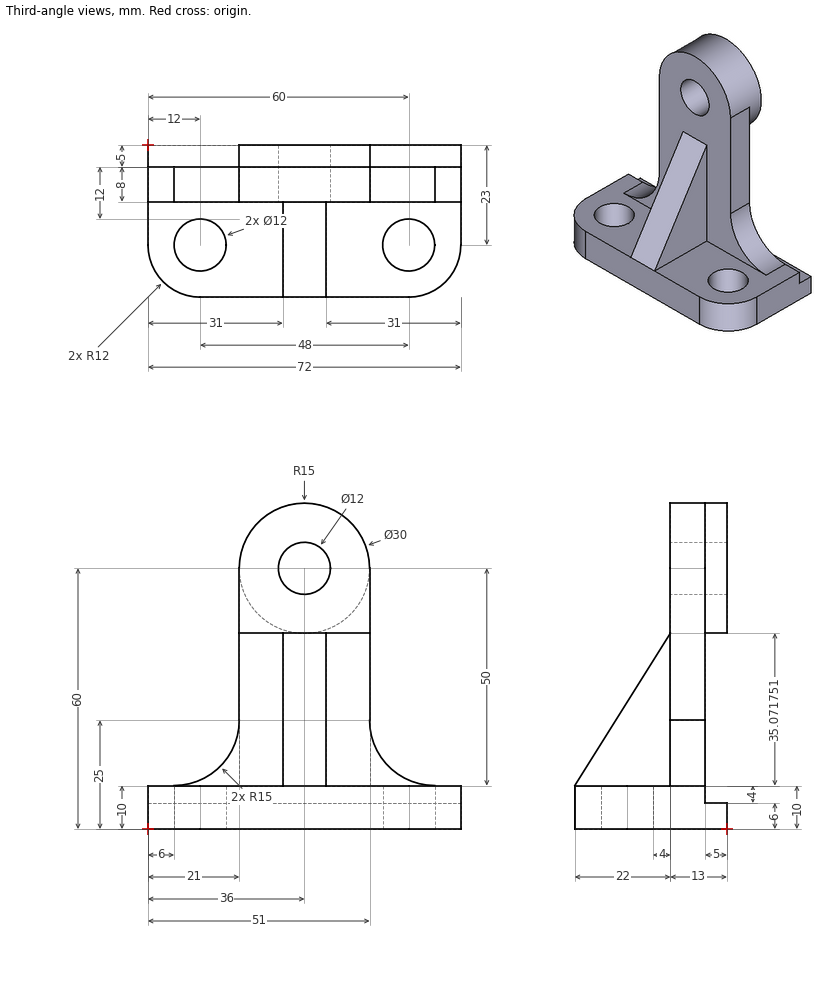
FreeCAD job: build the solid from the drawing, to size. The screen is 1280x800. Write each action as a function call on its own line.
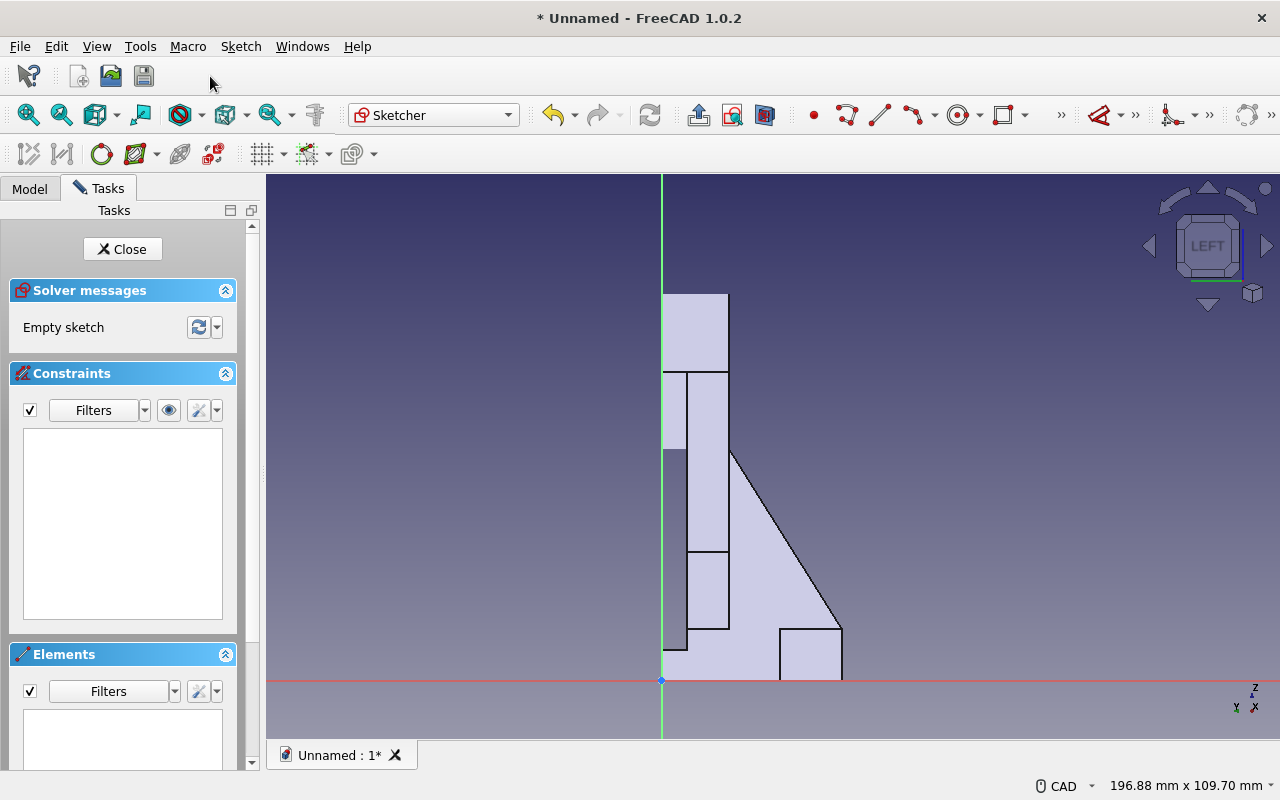
scroll(848, 711, up, 2)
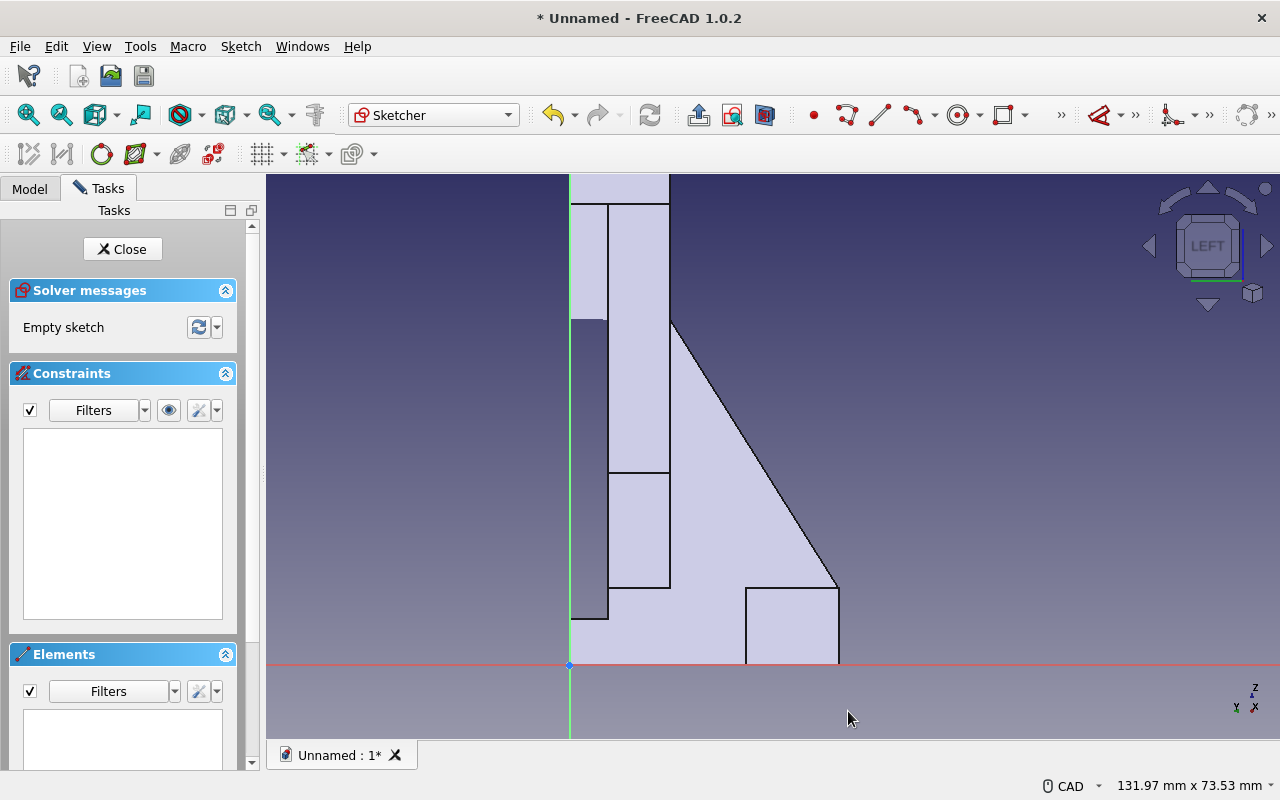
click(847, 116)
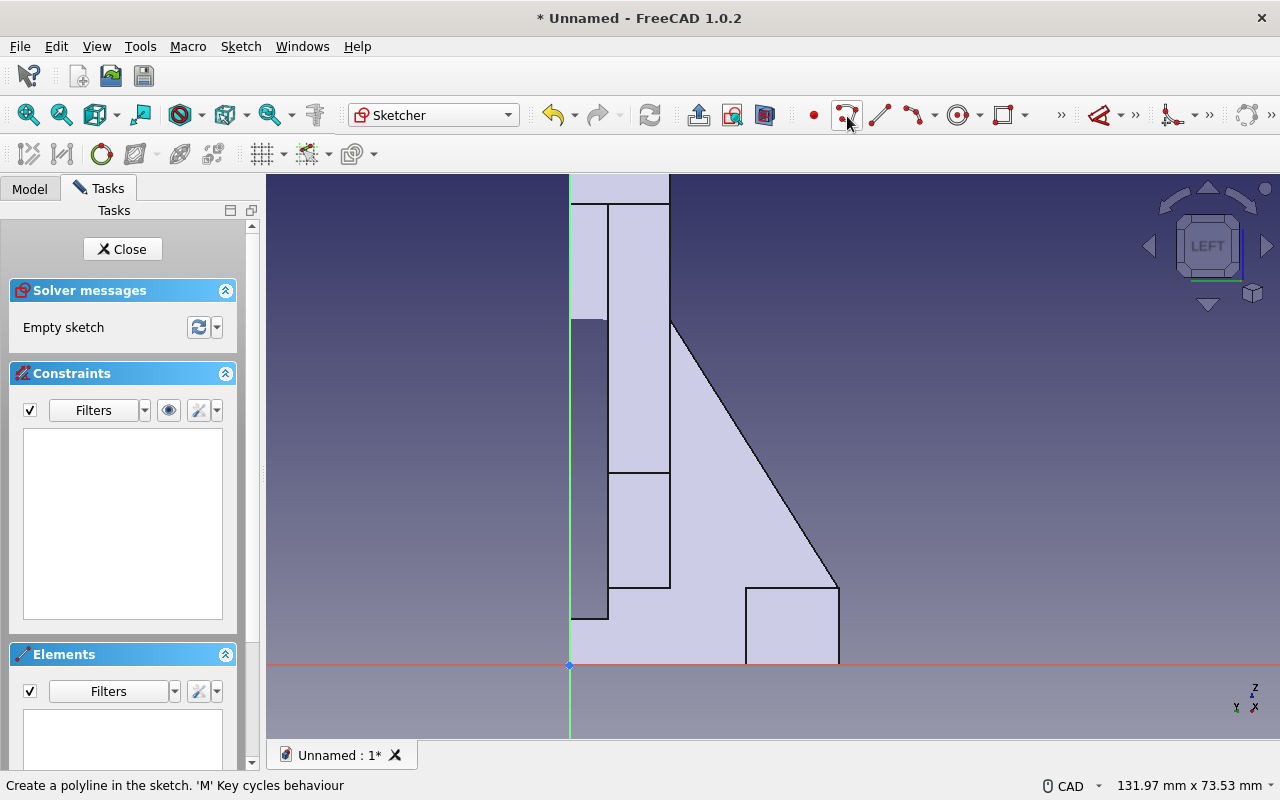
click(670, 588)
click(839, 588)
click(670, 319)
click(670, 589)
key(Escape)
key(Escape)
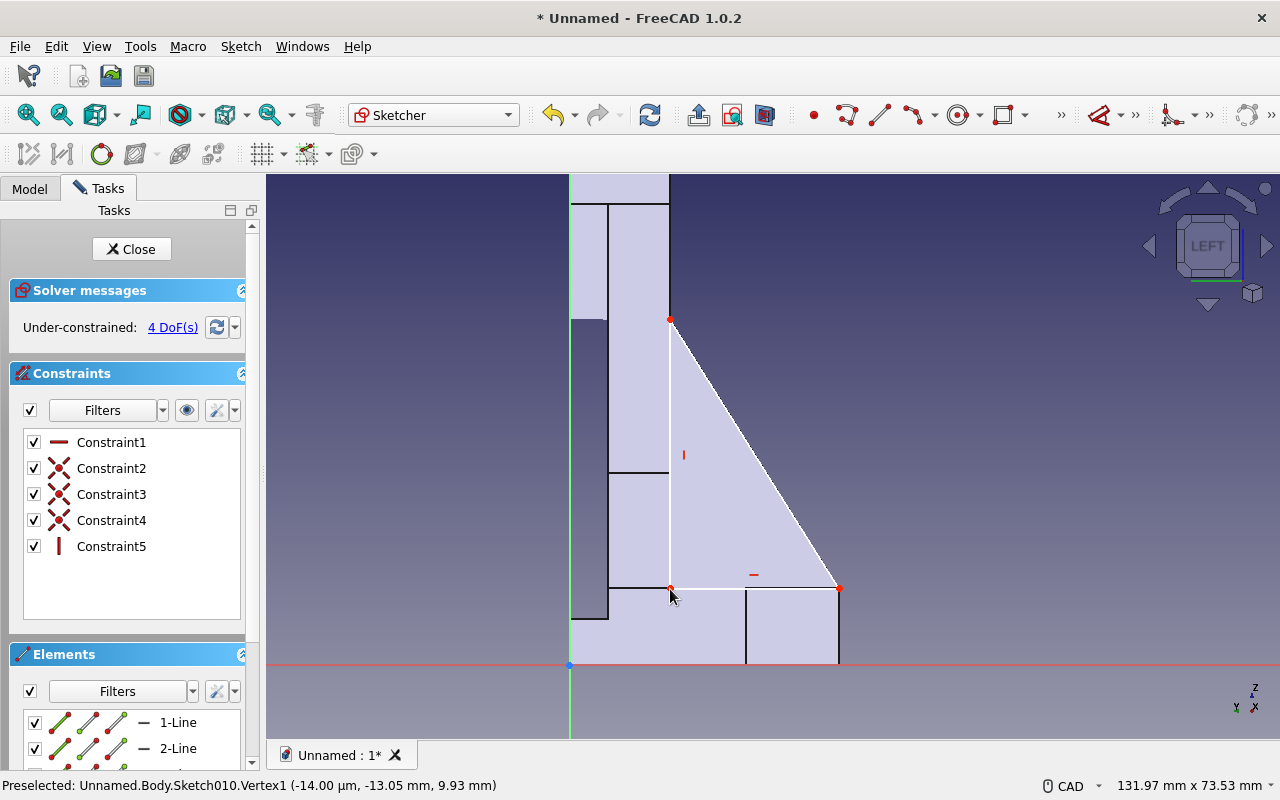
click(1098, 116)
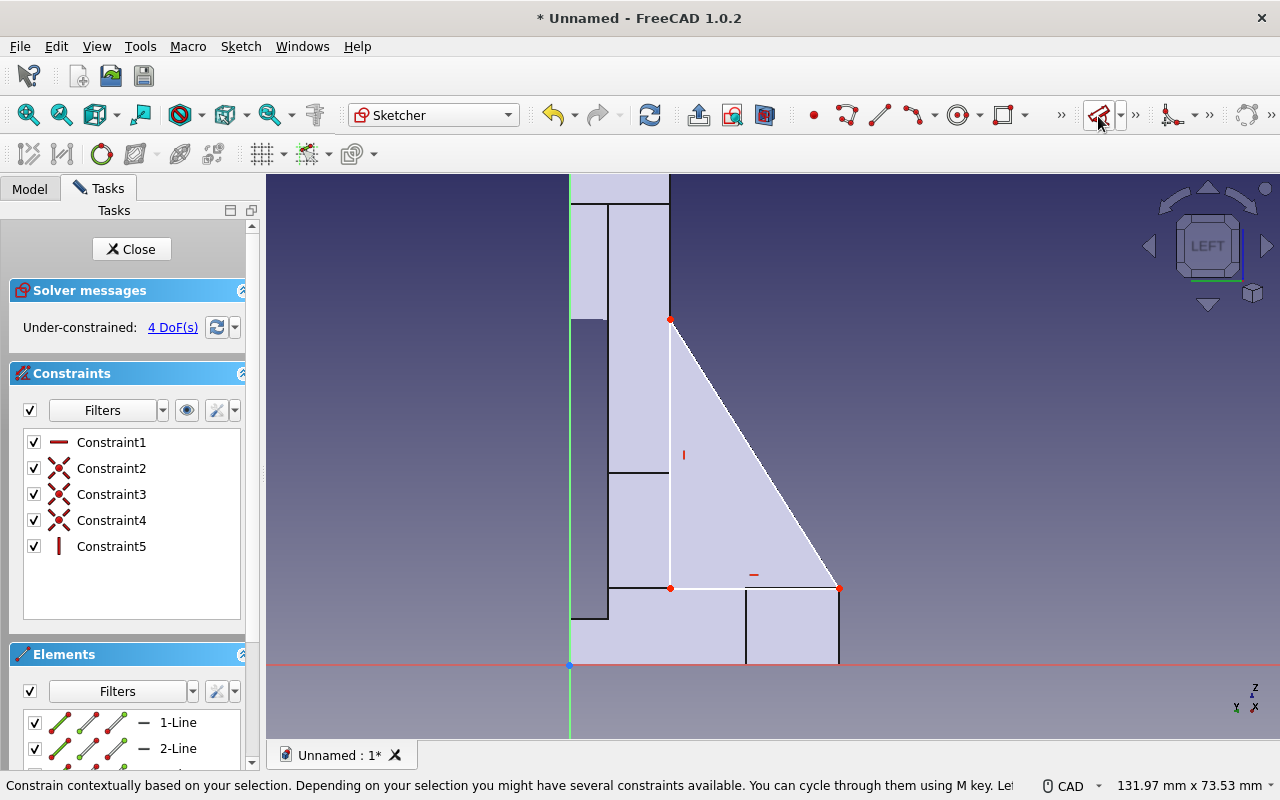
click(721, 589)
click(754, 623)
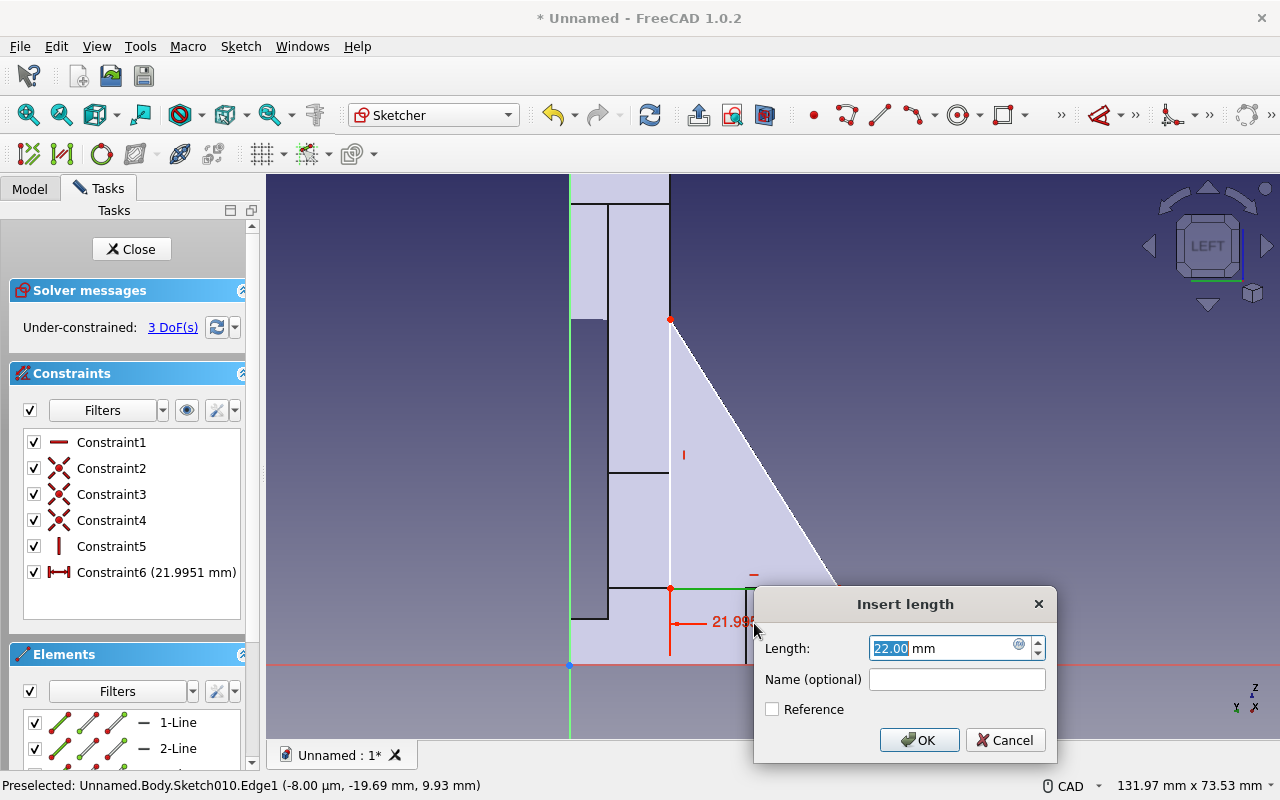
text(22)
key(Return)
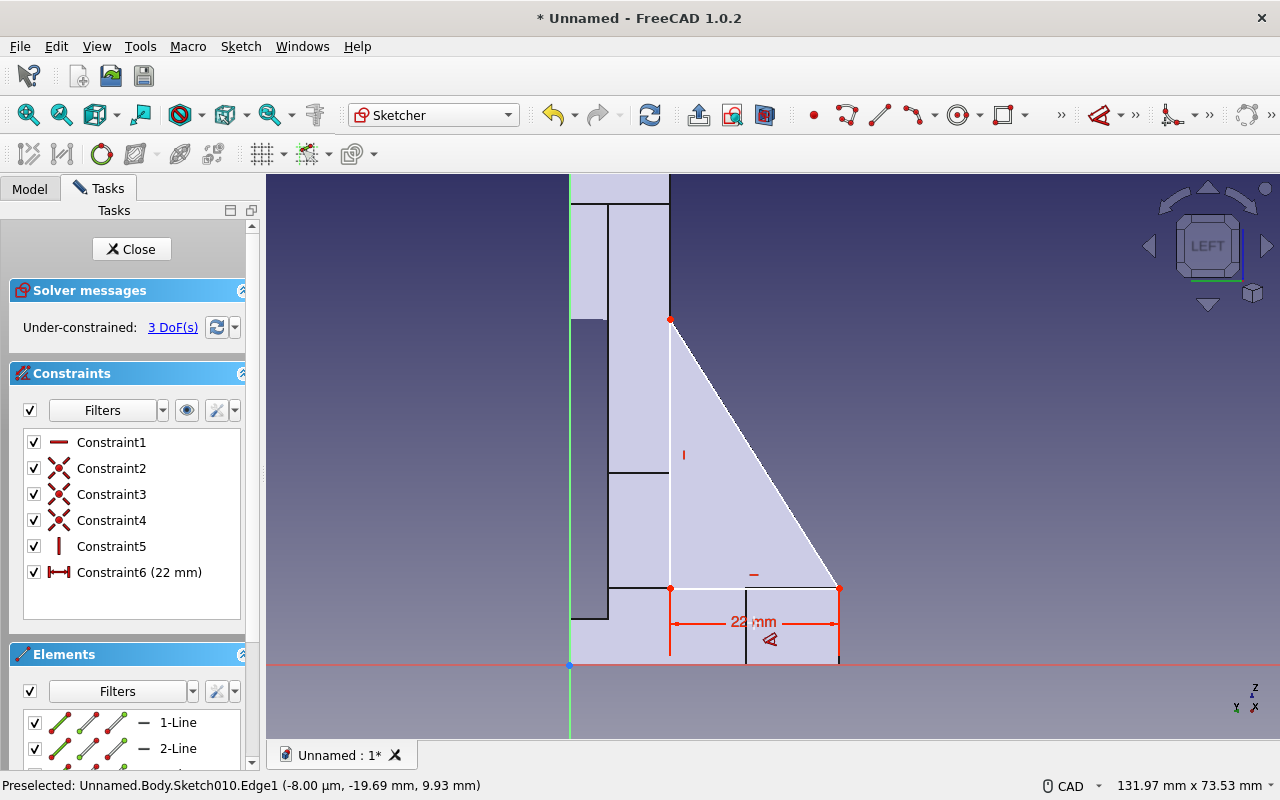
click(670, 589)
click(620, 699)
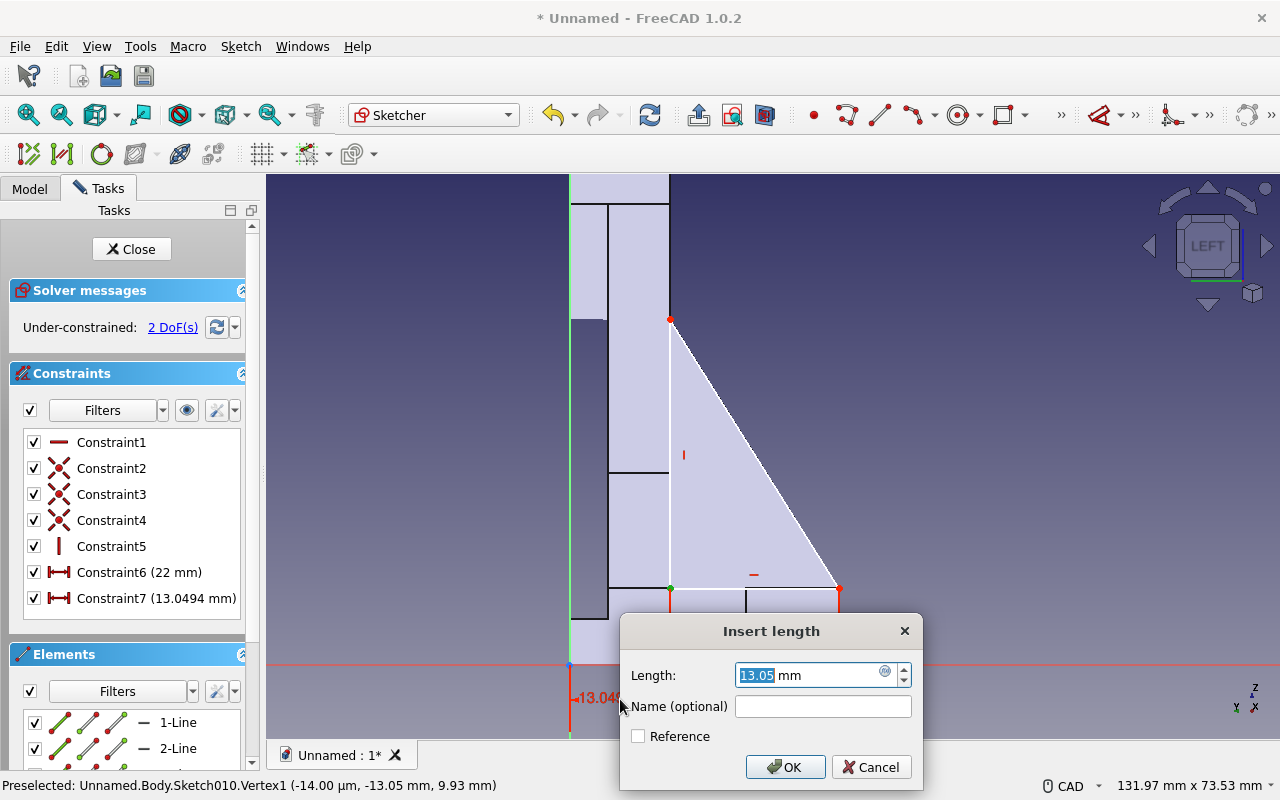
text(13)
key(Return)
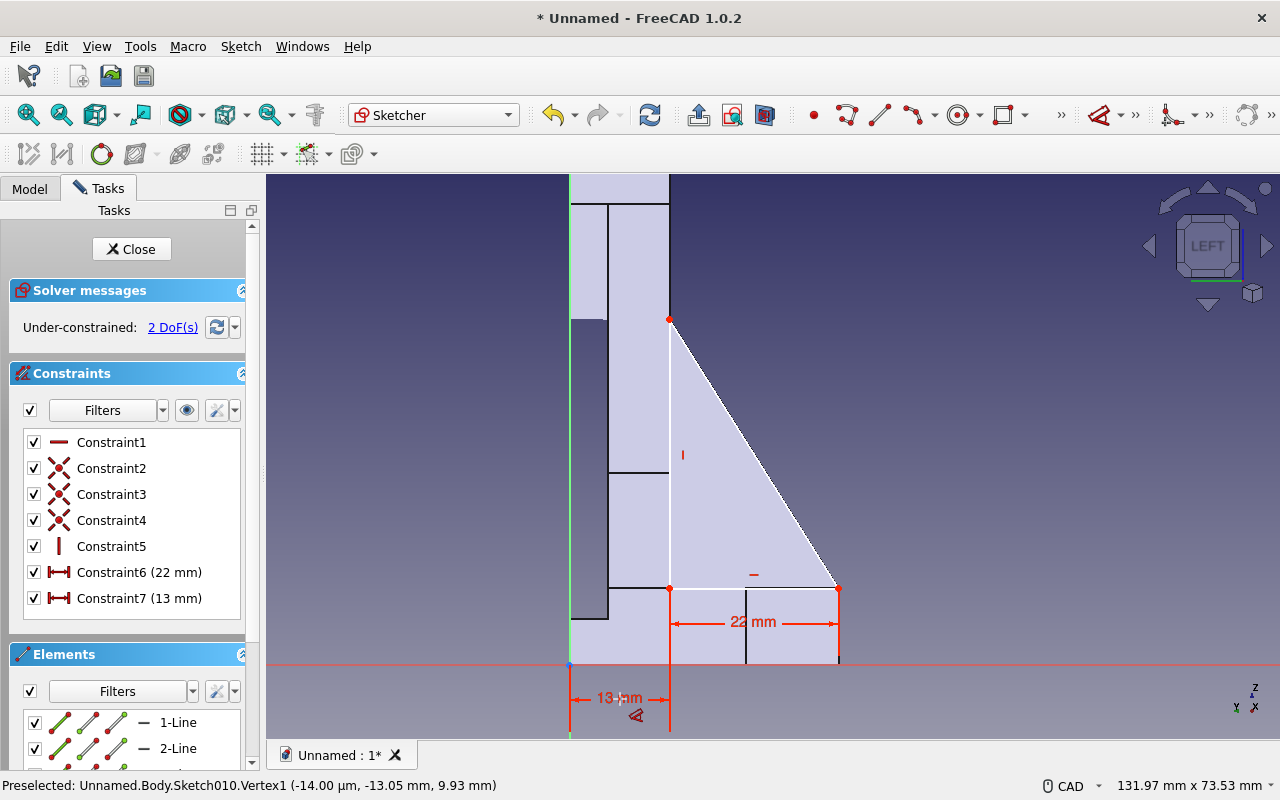
click(670, 589)
click(536, 627)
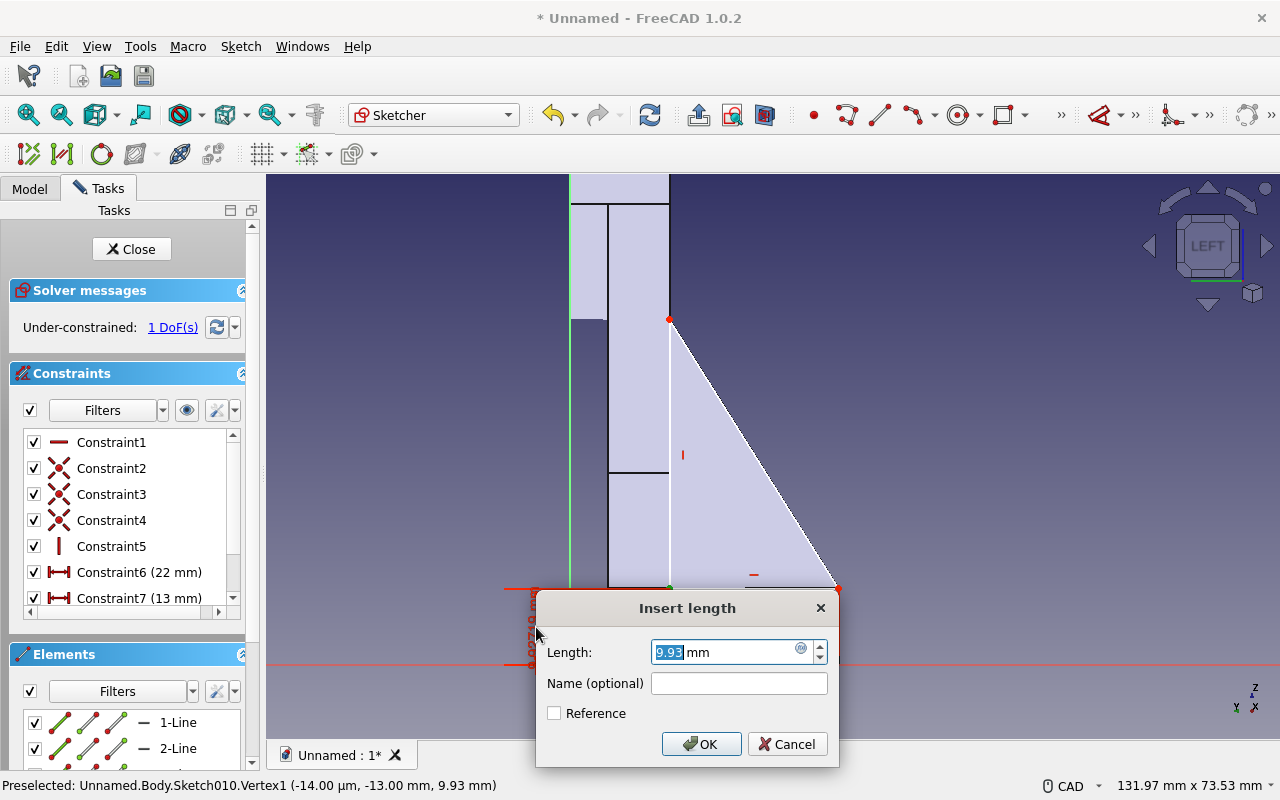
text(10)
key(Return)